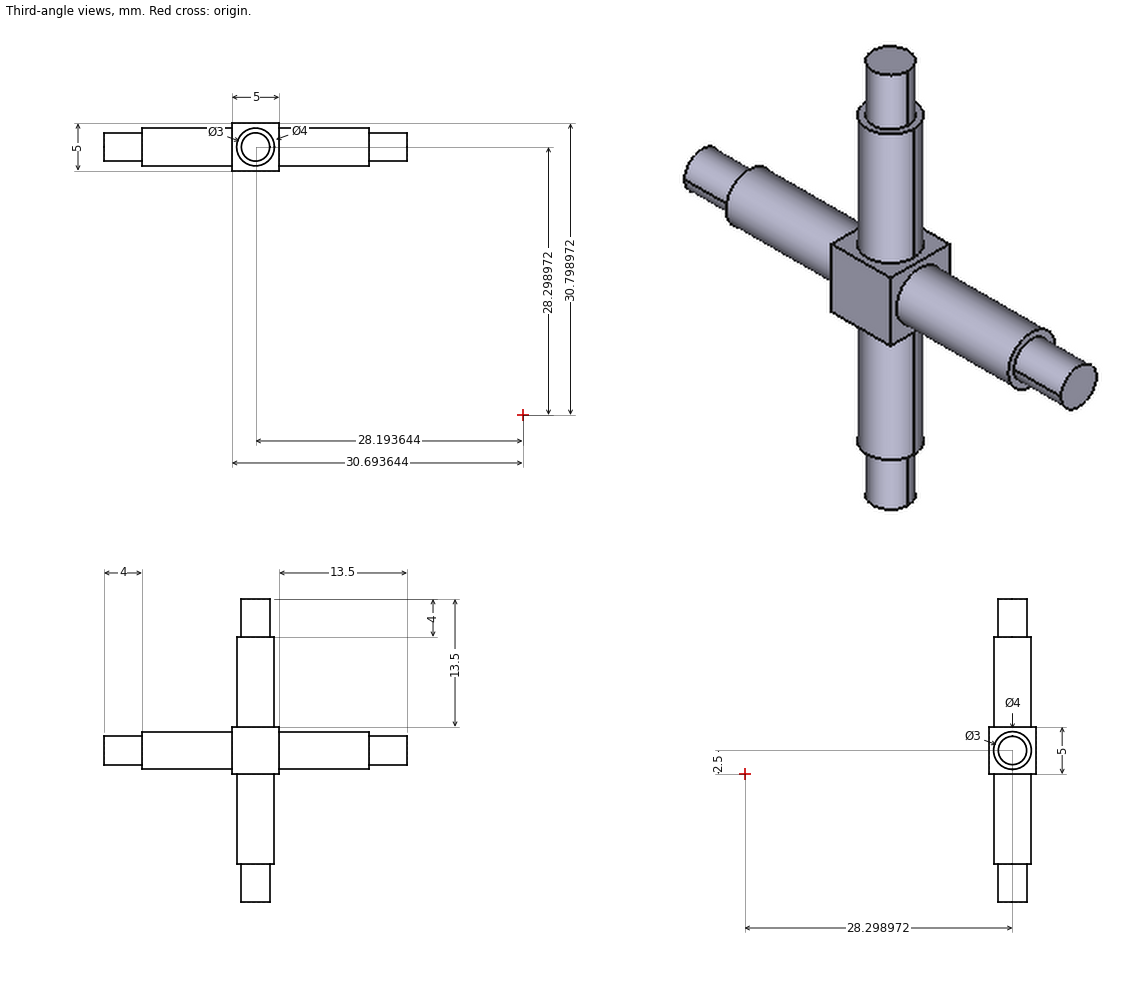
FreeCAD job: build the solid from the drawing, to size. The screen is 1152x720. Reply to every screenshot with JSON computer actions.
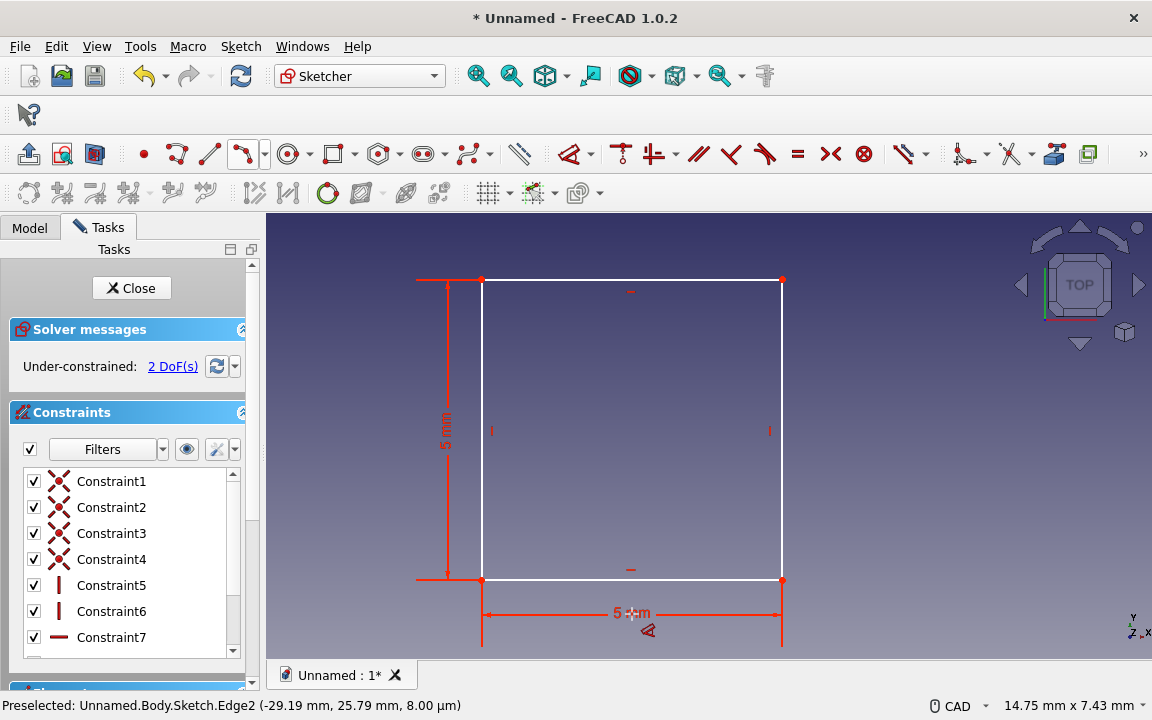
{"action": "left_click", "coordinate": [482, 280]}
{"action": "left_click", "coordinate": [734, 246]}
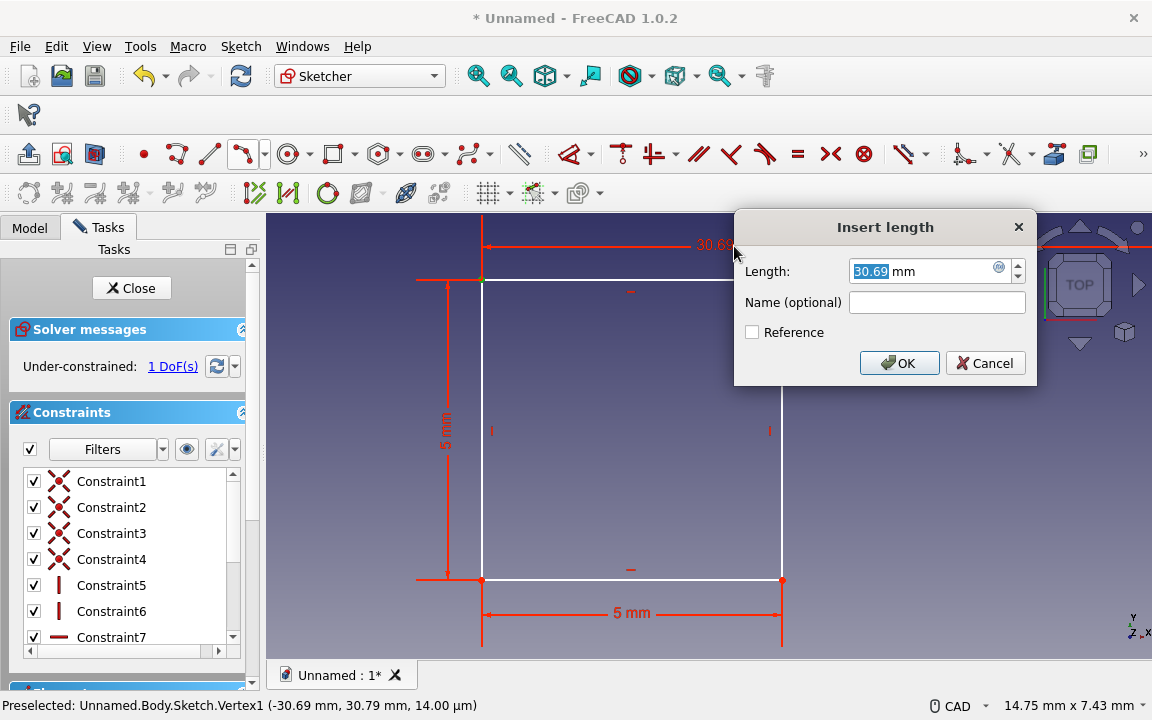
{"action": "type", "text": "30.693644"}
{"action": "key", "text": "Return"}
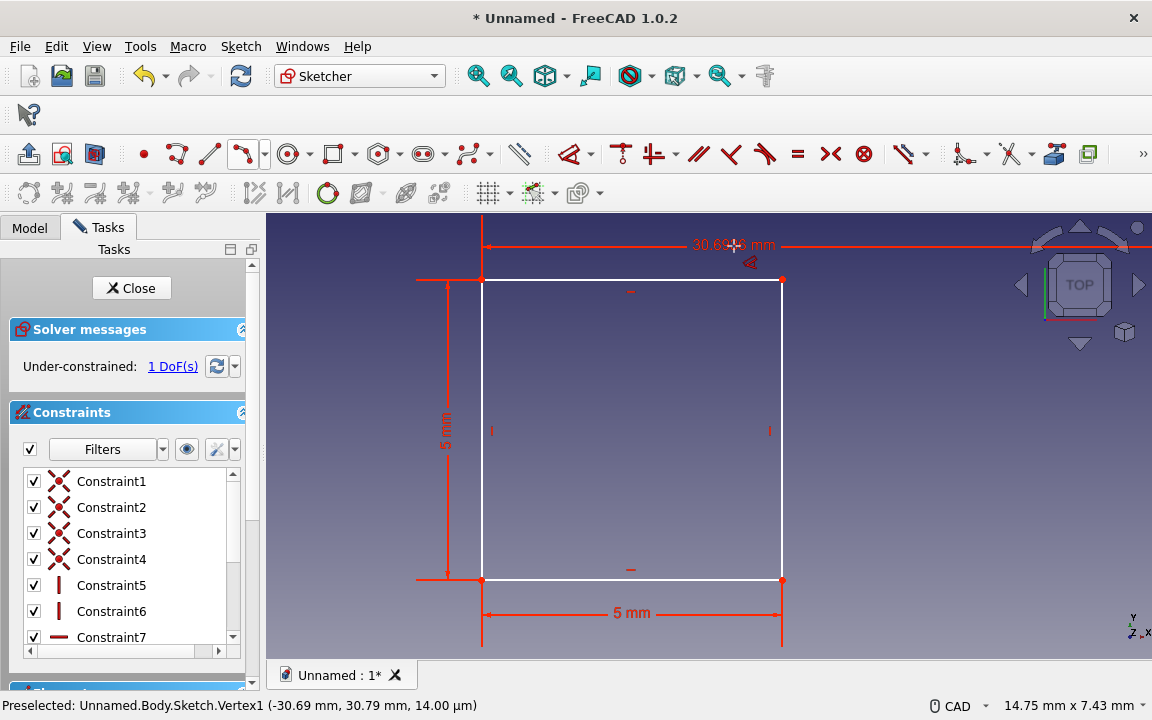
{"action": "left_click", "coordinate": [482, 280]}
{"action": "left_click", "coordinate": [448, 456]}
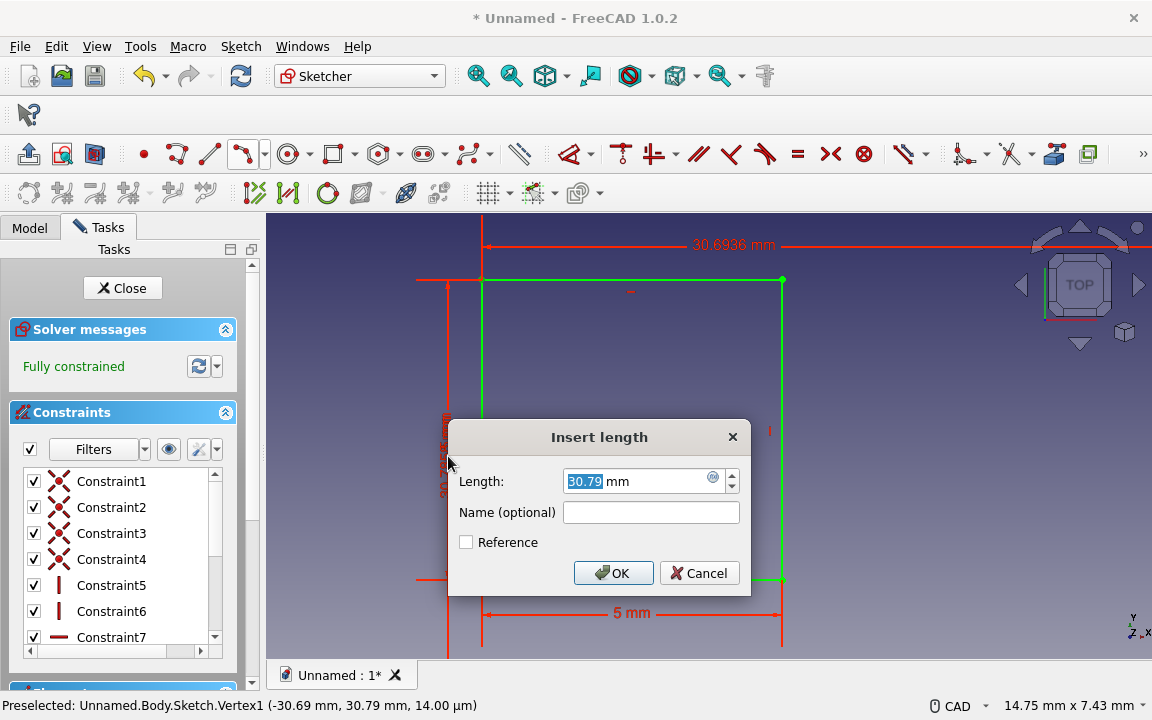
{"action": "type", "text": "30.798972"}
{"action": "key", "text": "Return"}
{"action": "key", "text": "Escape"}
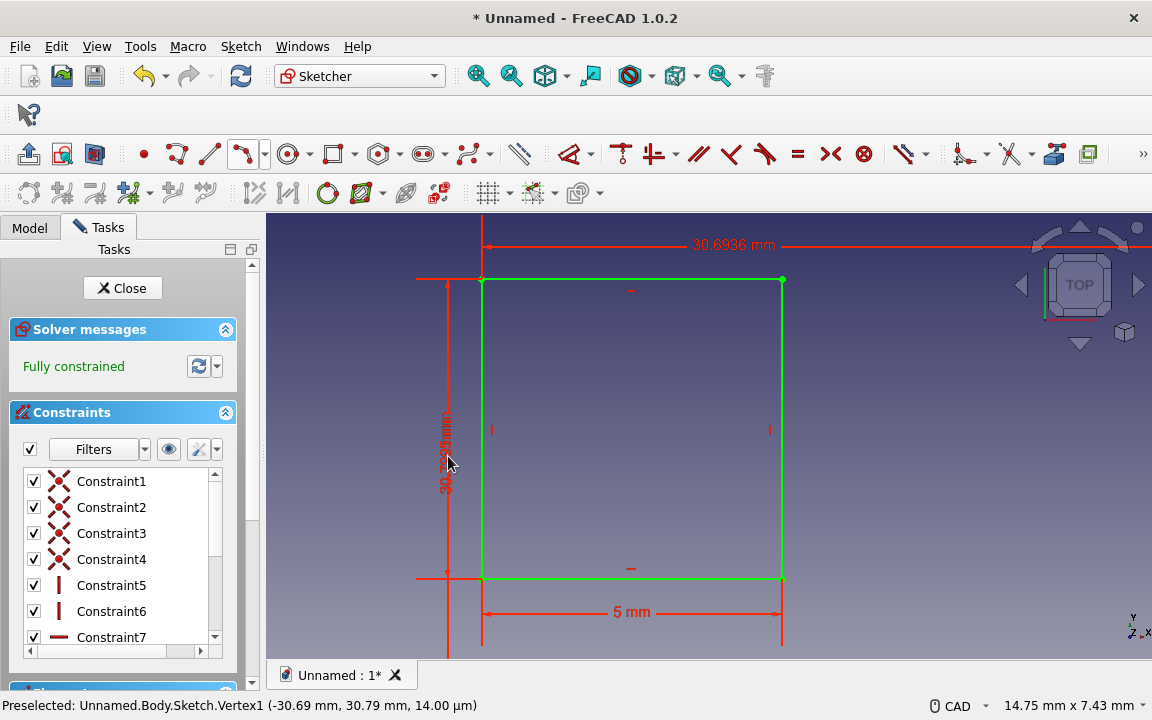
{"action": "left_click", "coordinate": [123, 288]}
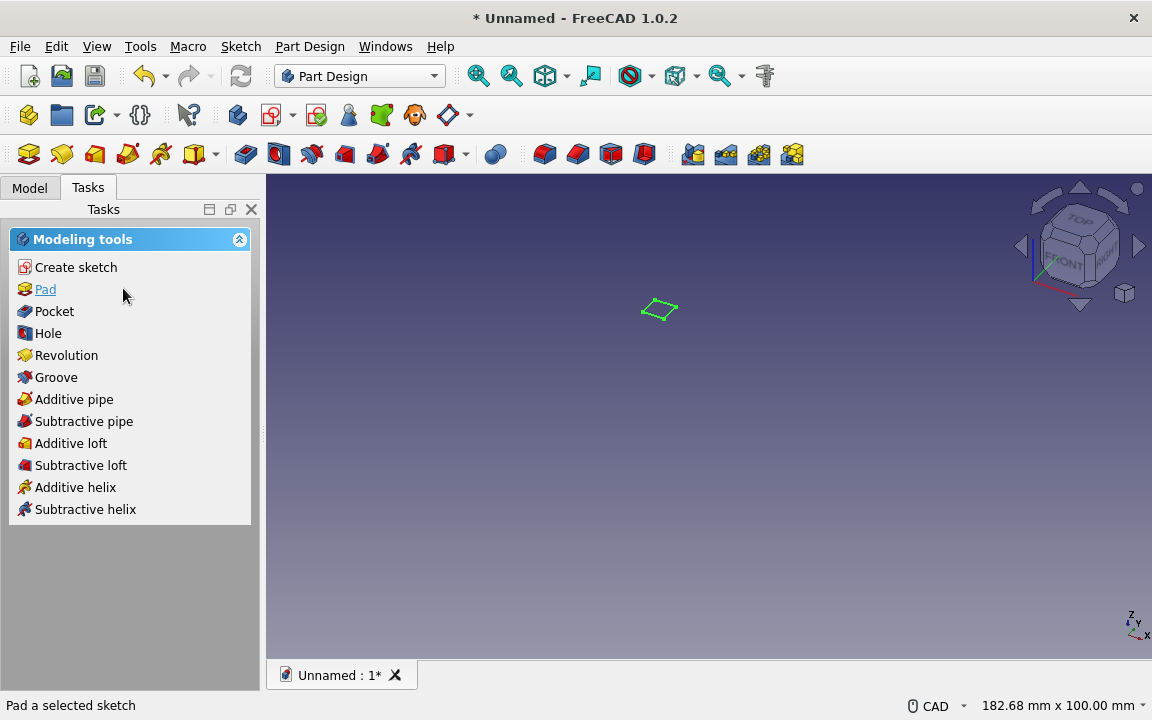
{"action": "left_click", "coordinate": [29, 154]}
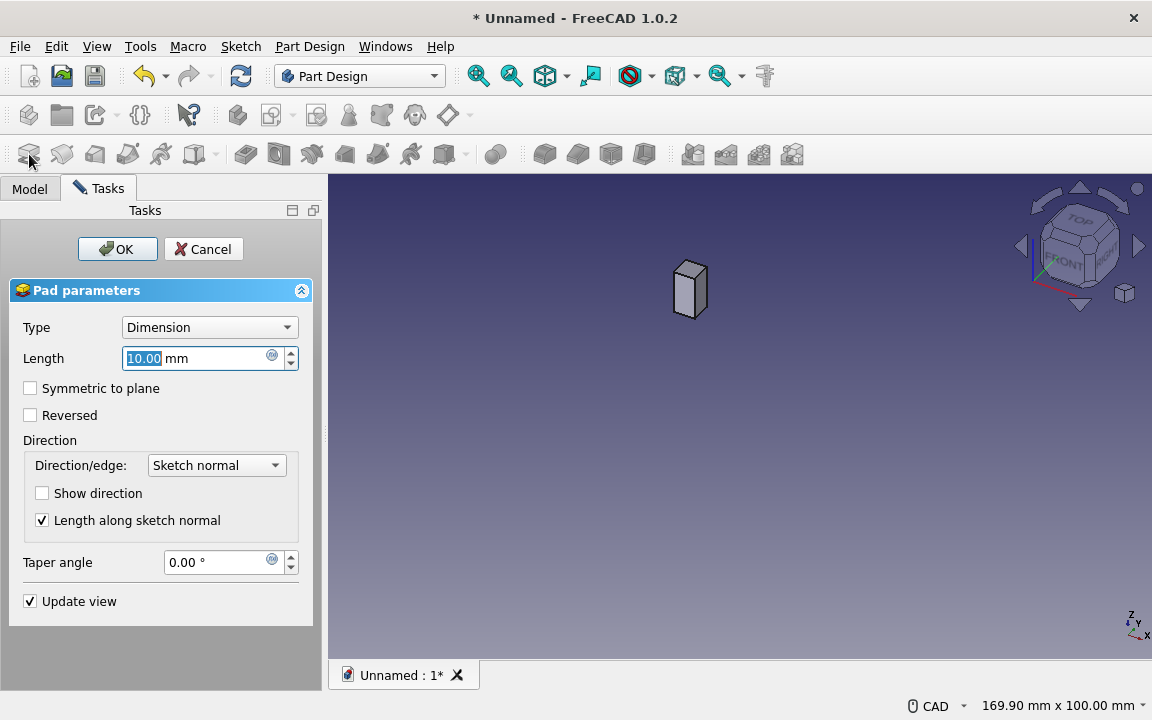
{"action": "type", "text": "5"}
{"action": "key", "text": "Tab"}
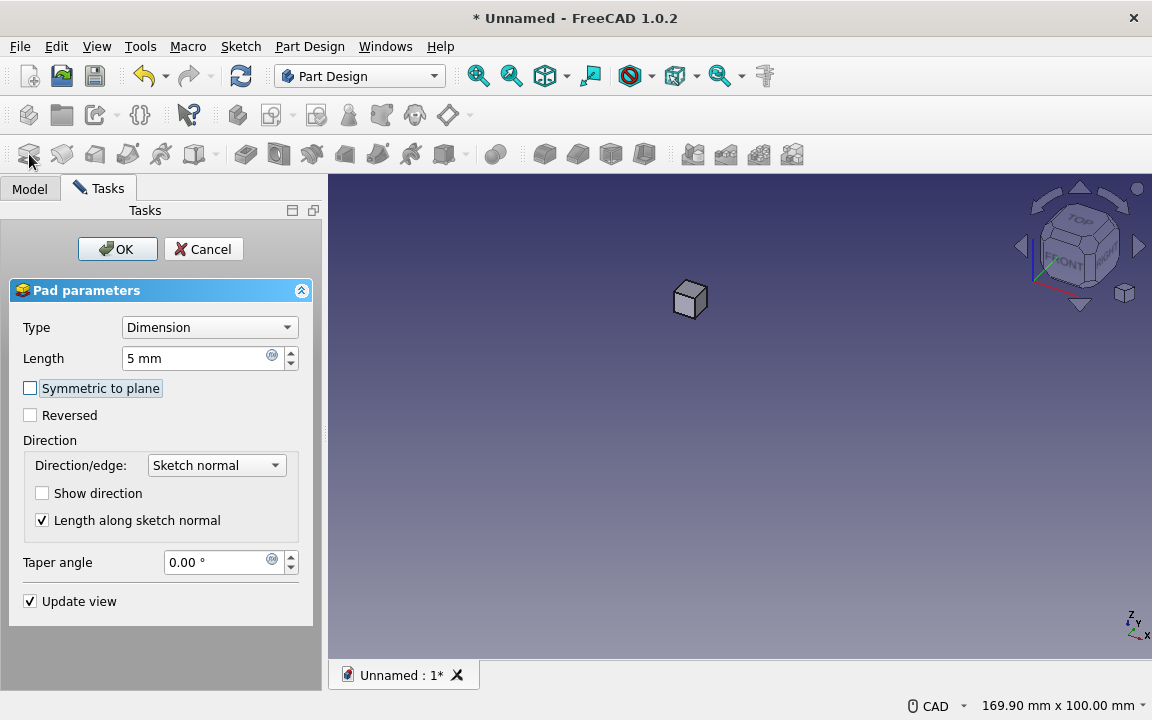
{"action": "left_click", "coordinate": [118, 249]}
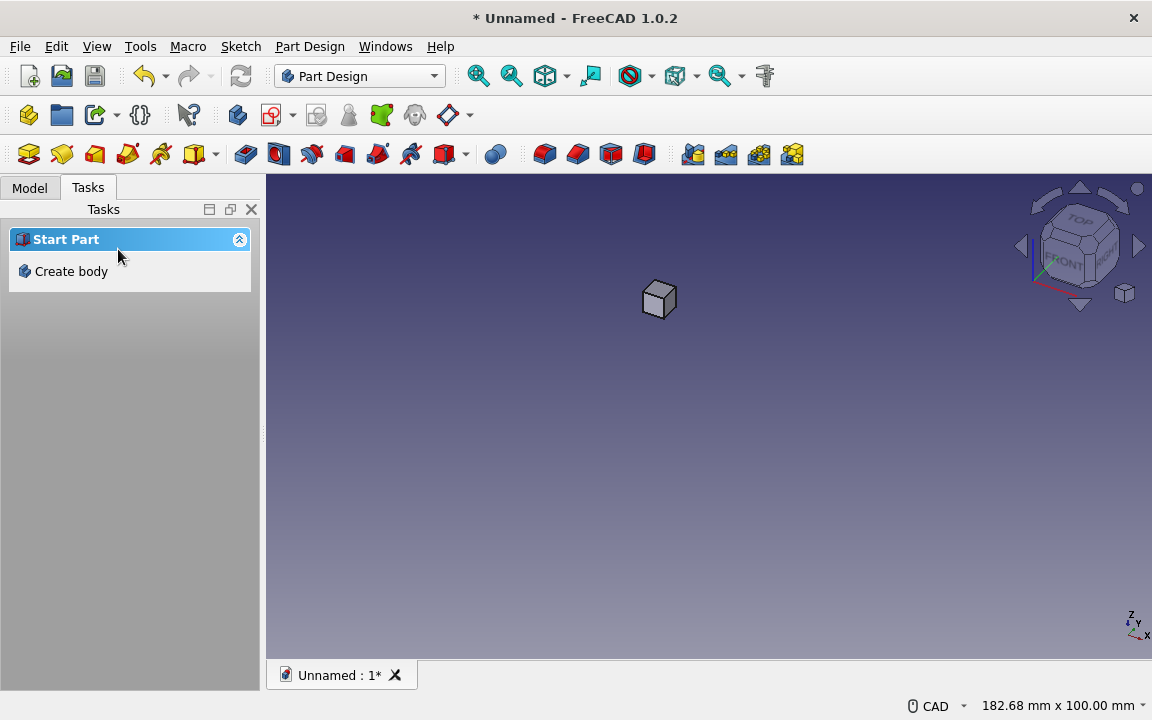
{"action": "key", "text": "v f"}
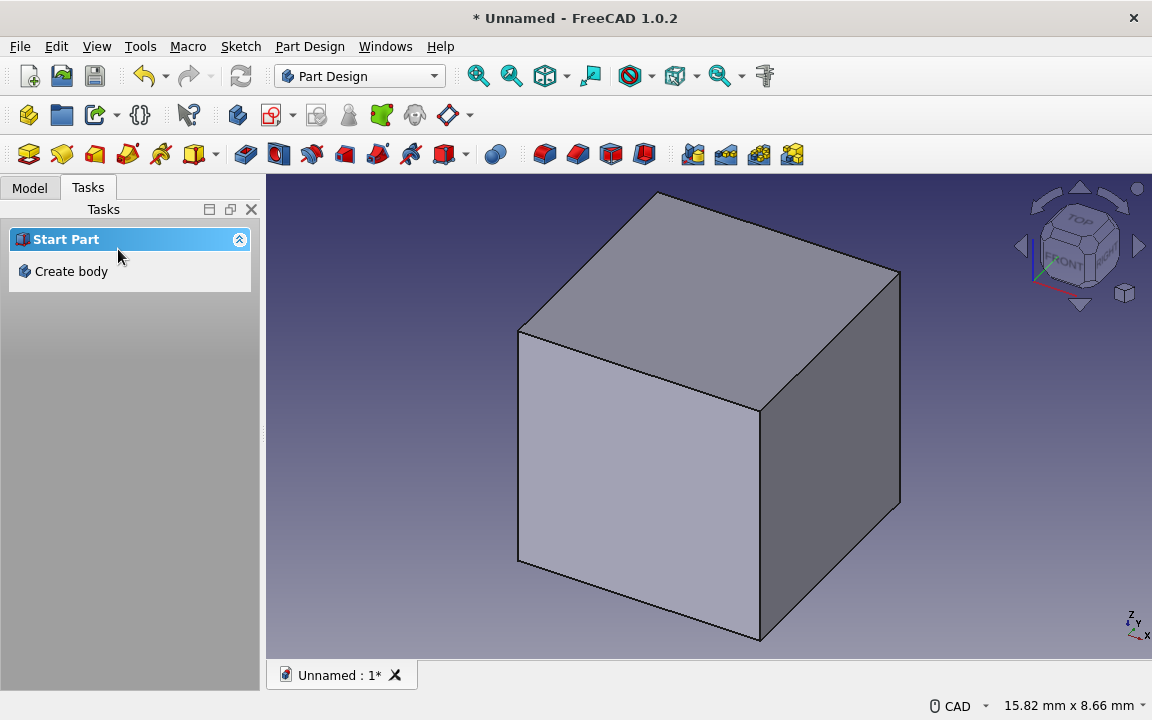
{"action": "left_click", "coordinate": [709, 301]}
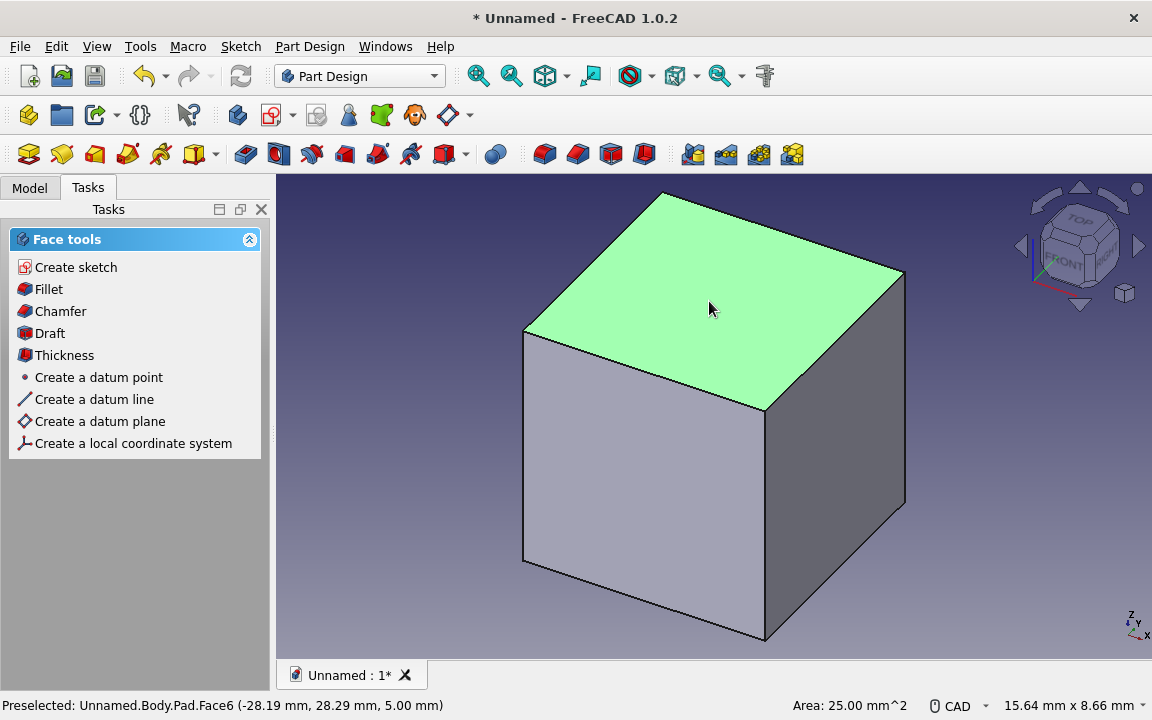
{"action": "left_click", "coordinate": [270, 116]}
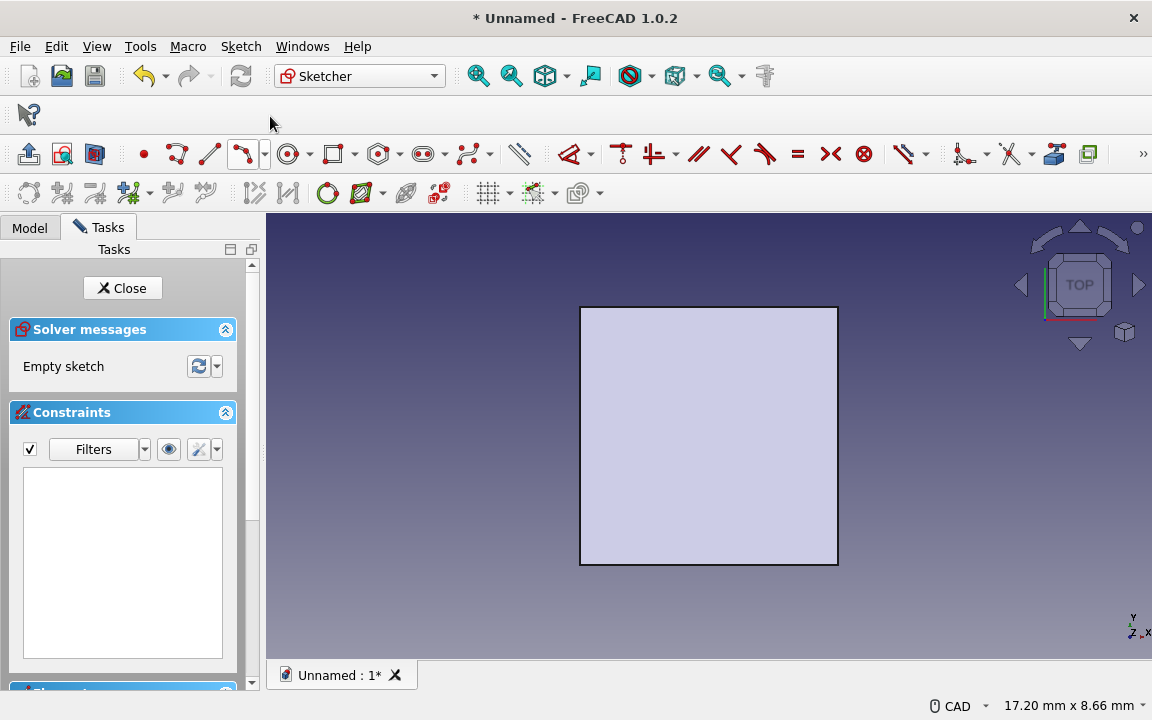
{"action": "key", "text": "g c"}